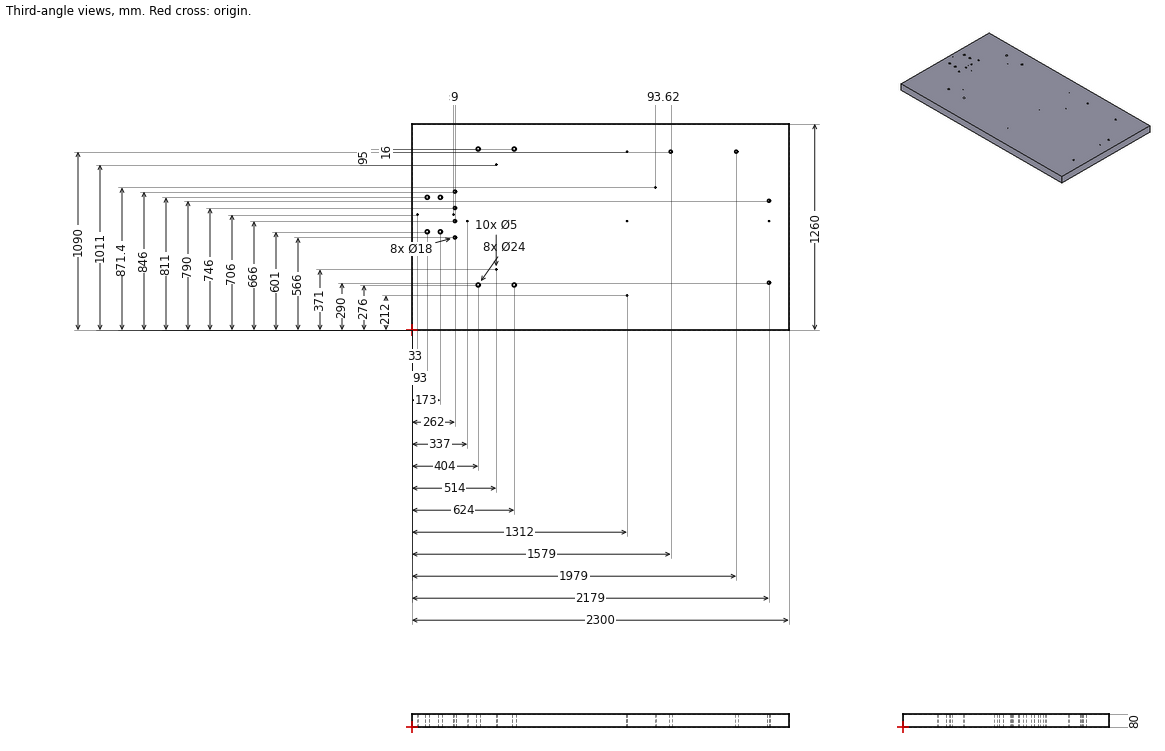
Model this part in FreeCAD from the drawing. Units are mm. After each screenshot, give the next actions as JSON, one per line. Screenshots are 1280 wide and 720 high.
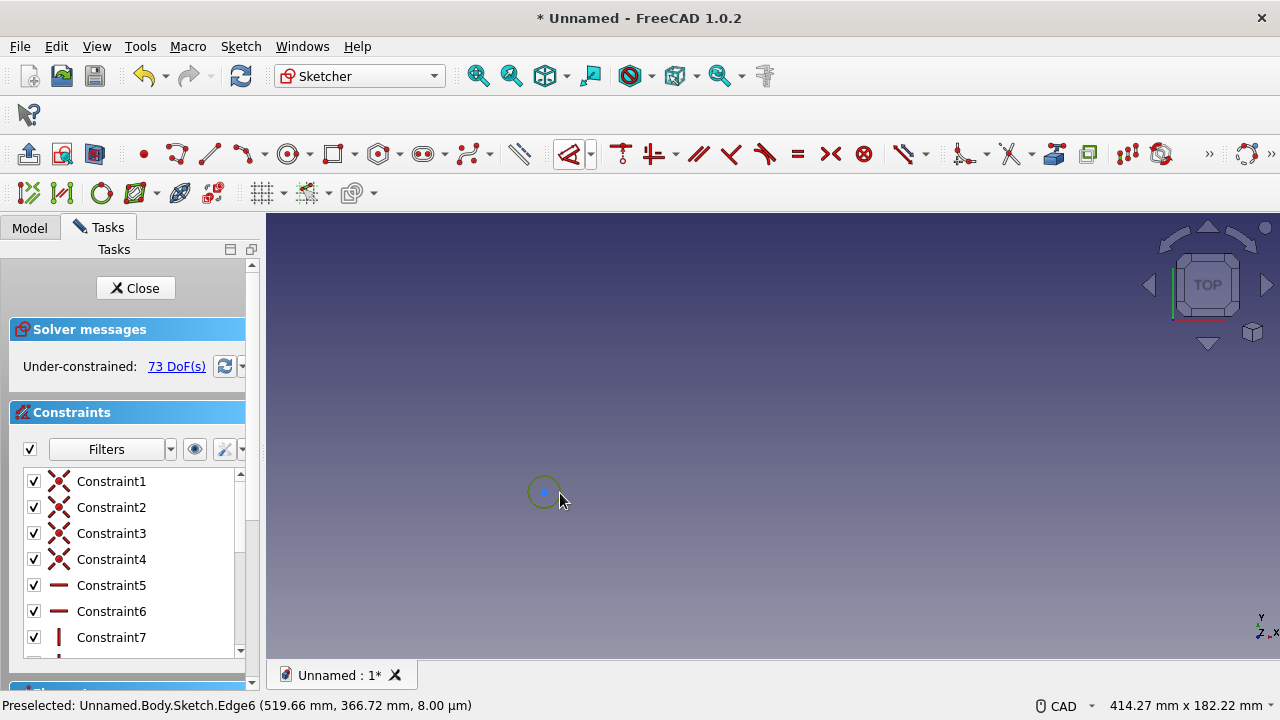
{"action": "scroll", "coordinate": [565, 495], "scroll_direction": "down", "scroll_amount": 12}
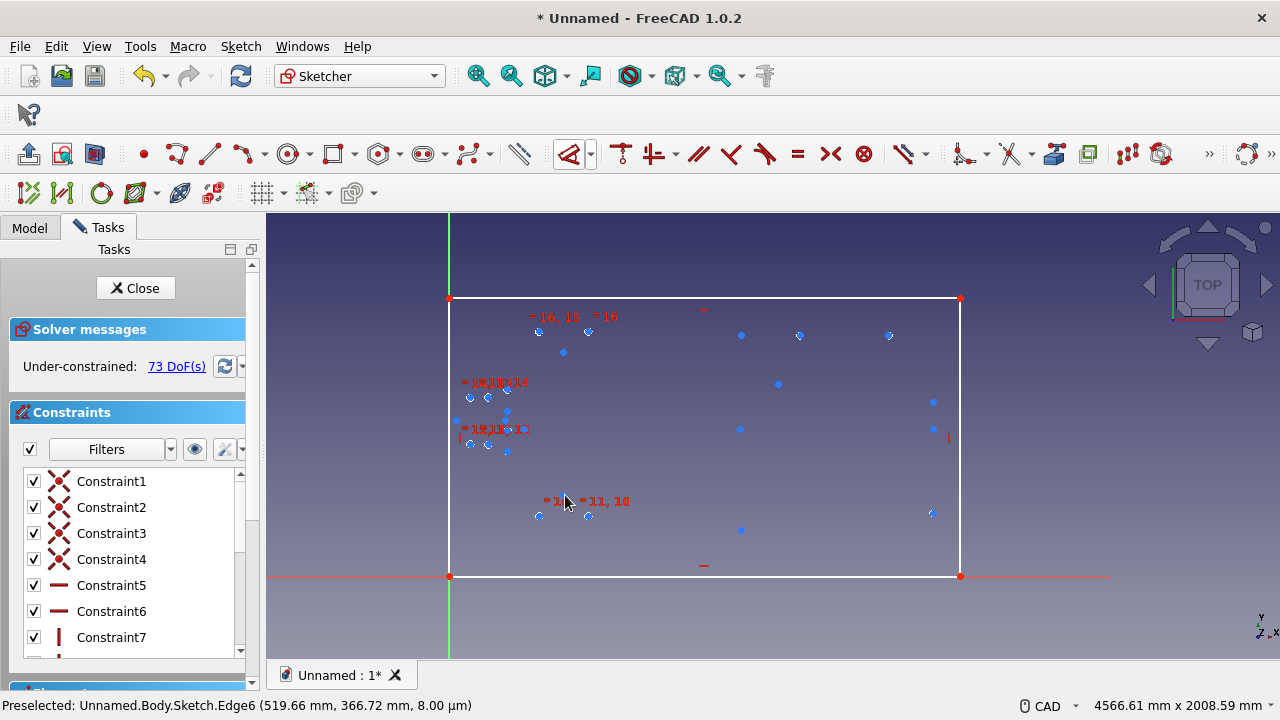
{"action": "scroll", "coordinate": [742, 530], "scroll_direction": "up", "scroll_amount": 14}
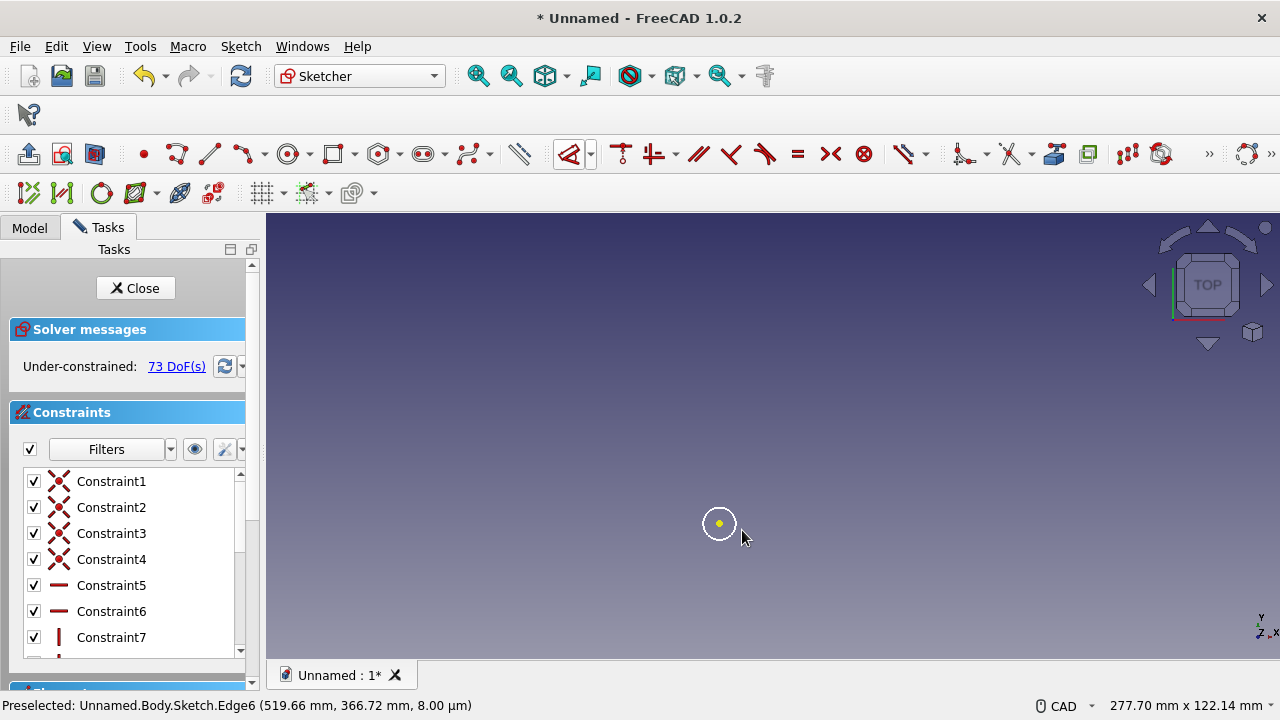
{"action": "left_click", "coordinate": [731, 512]}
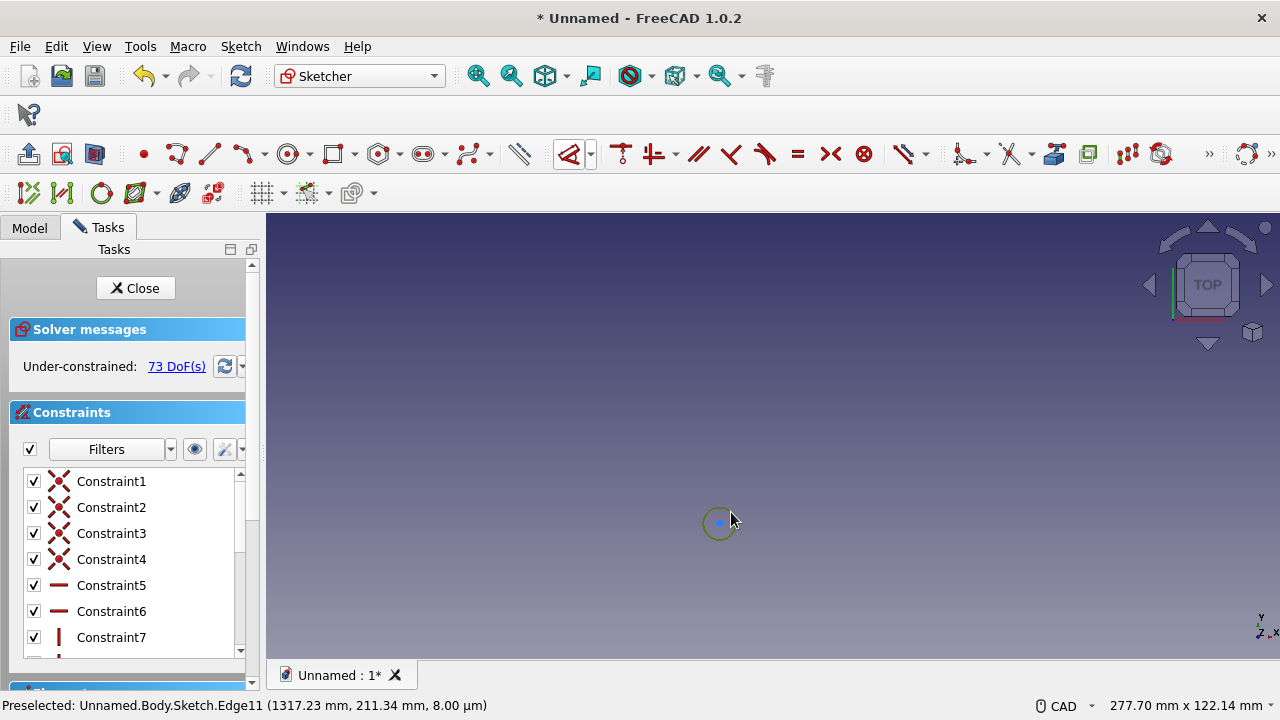
{"action": "scroll", "coordinate": [742, 530], "scroll_direction": "down", "scroll_amount": 14}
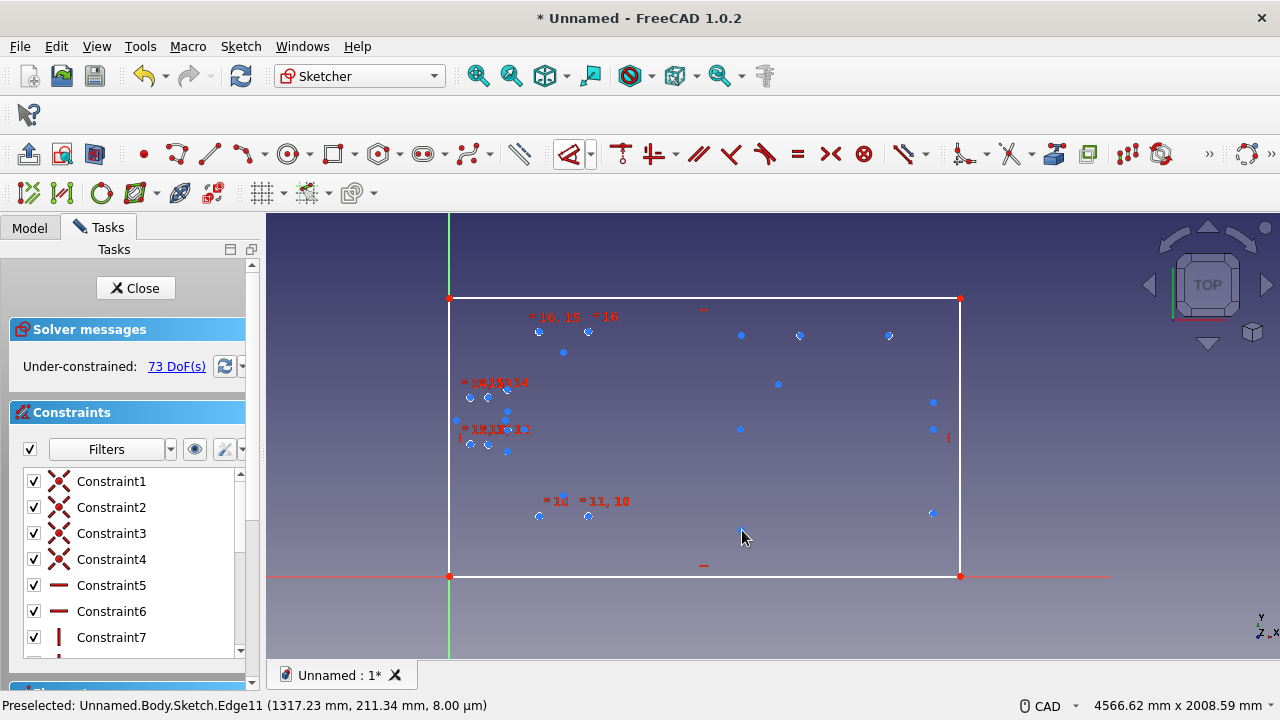
{"action": "scroll", "coordinate": [457, 420], "scroll_direction": "up", "scroll_amount": 14}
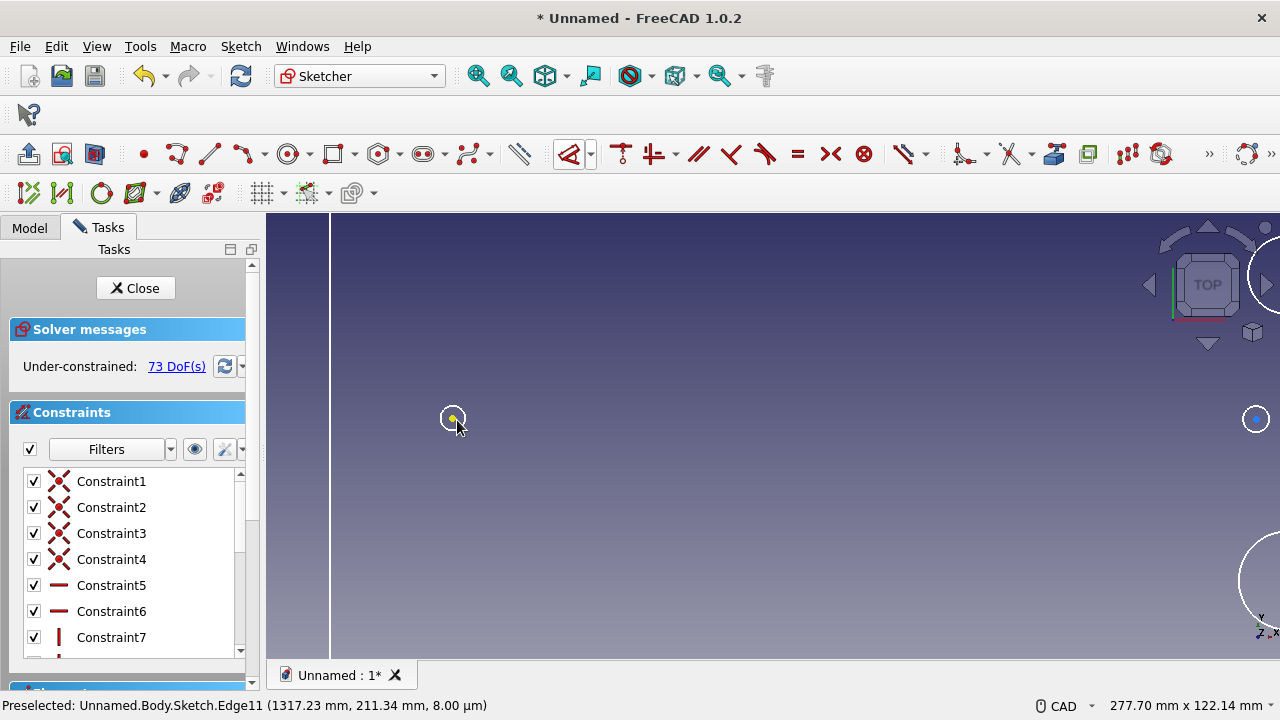
{"action": "left_click", "coordinate": [461, 409]}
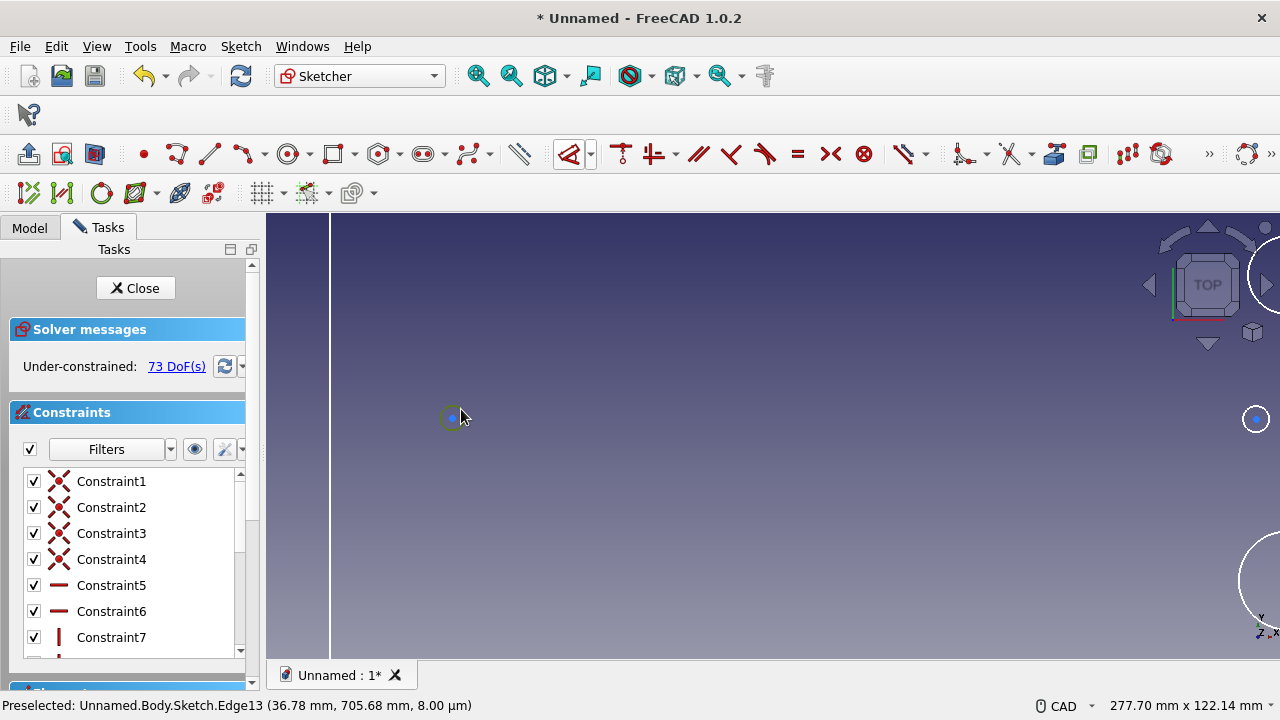
{"action": "scroll", "coordinate": [457, 420], "scroll_direction": "down", "scroll_amount": 14}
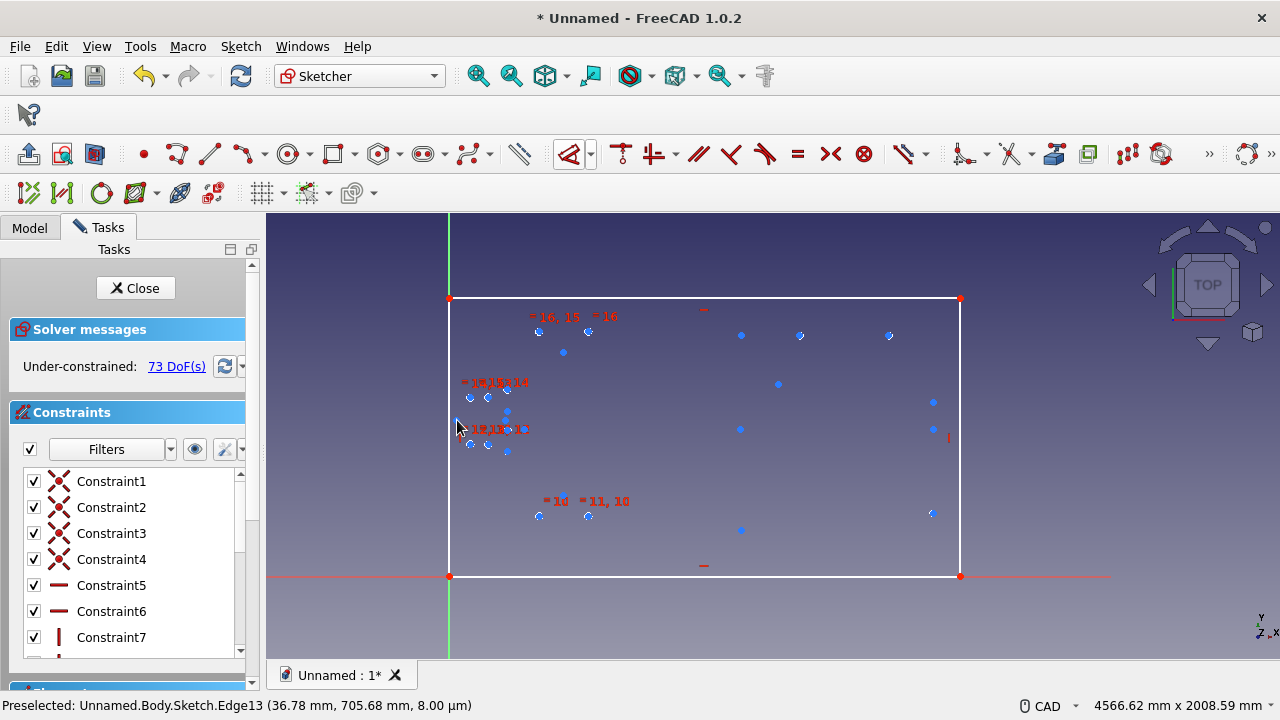
{"action": "scroll", "coordinate": [506, 420], "scroll_direction": "up", "scroll_amount": 14}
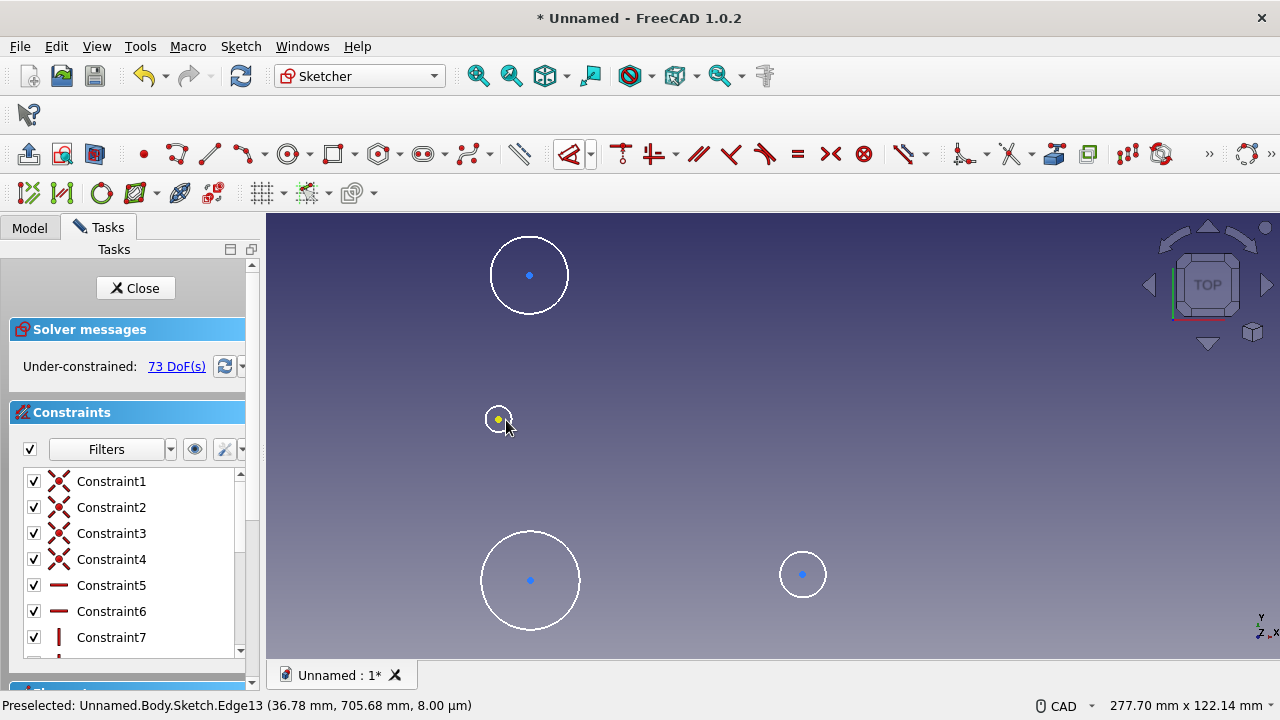
{"action": "left_click", "coordinate": [508, 410]}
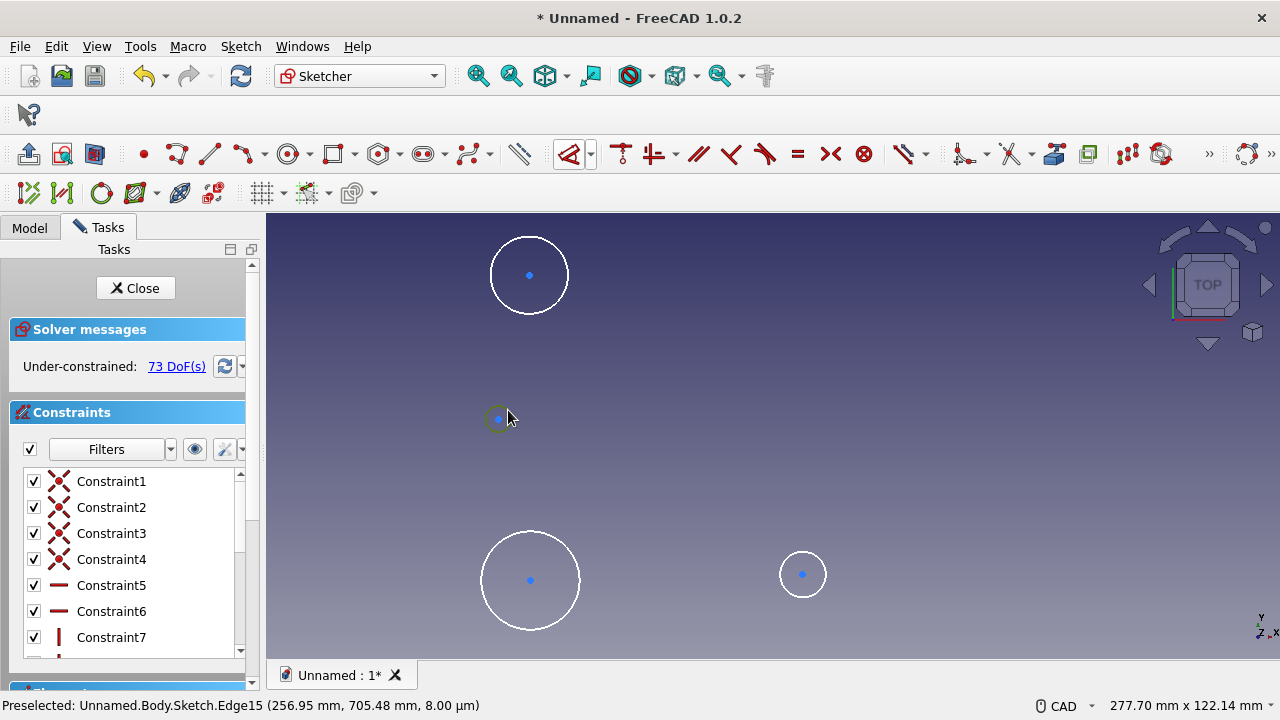
{"action": "left_click", "coordinate": [819, 558]}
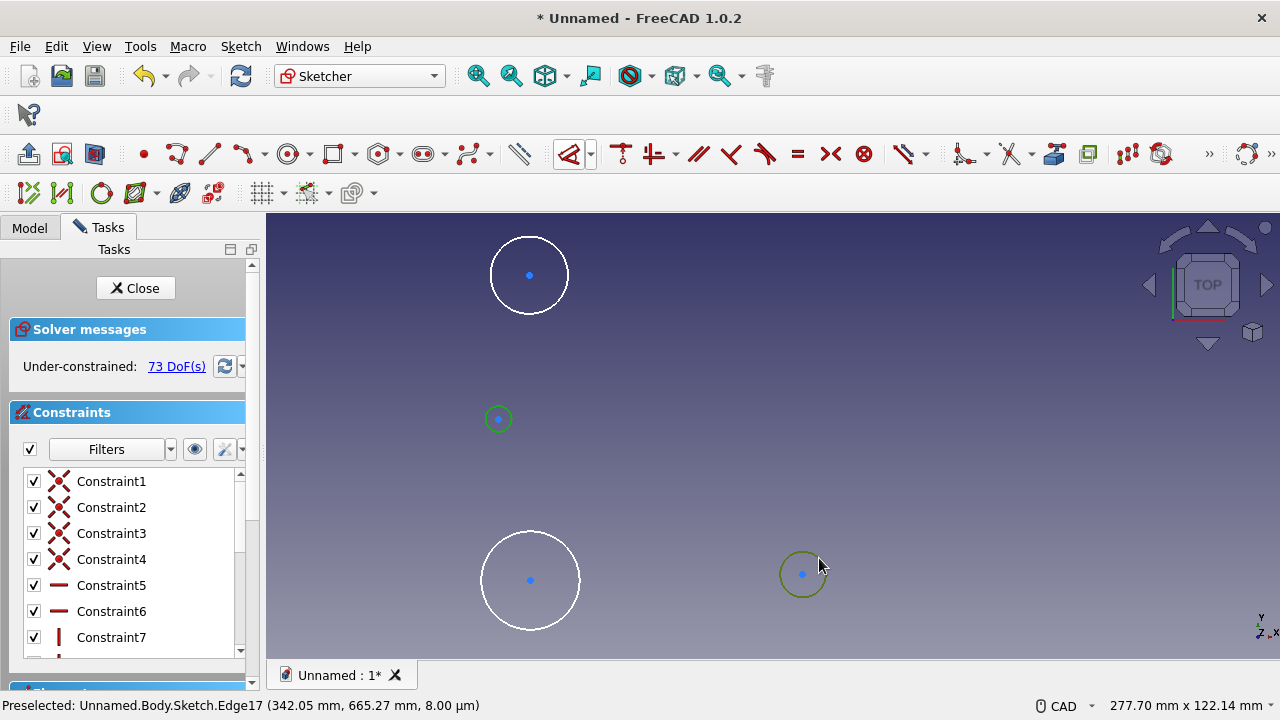
{"action": "scroll", "coordinate": [506, 420], "scroll_direction": "down", "scroll_amount": 14}